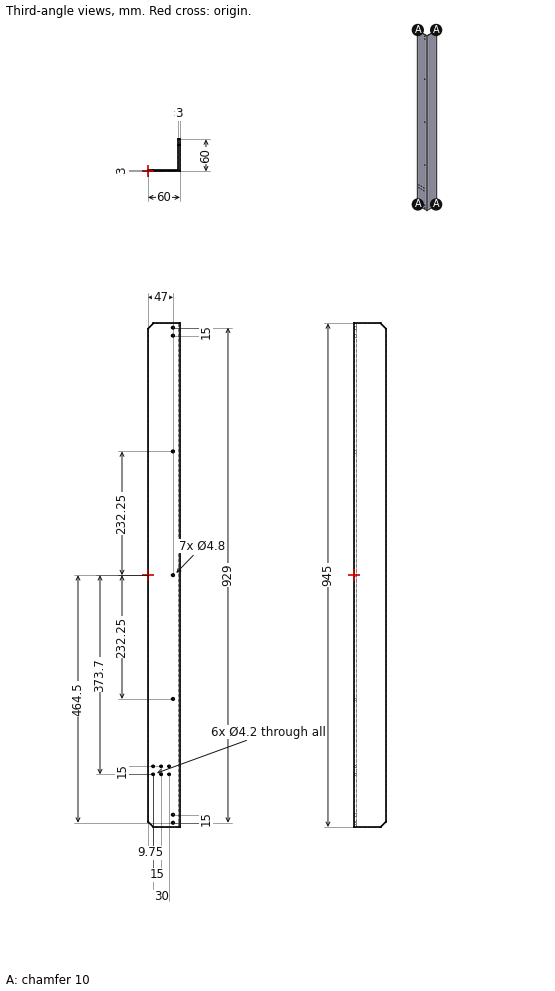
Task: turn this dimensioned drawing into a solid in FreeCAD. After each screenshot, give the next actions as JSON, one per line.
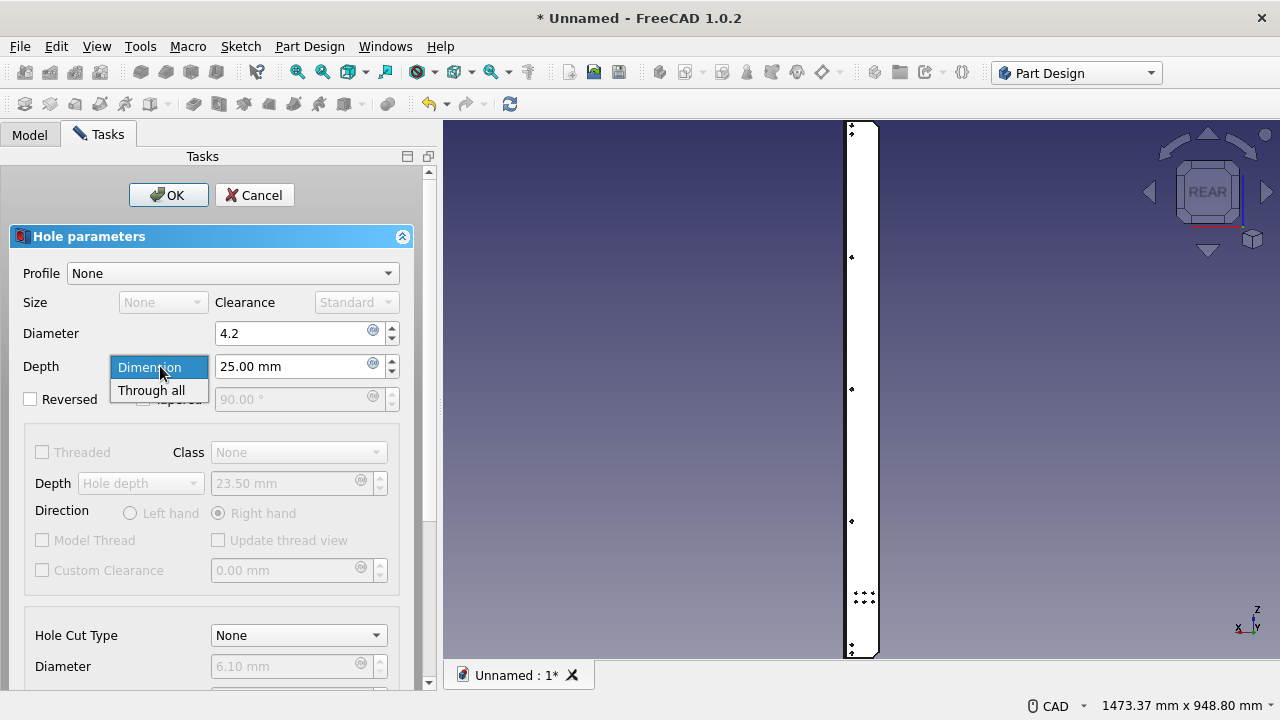
{"action": "left_click", "coordinate": [158, 390]}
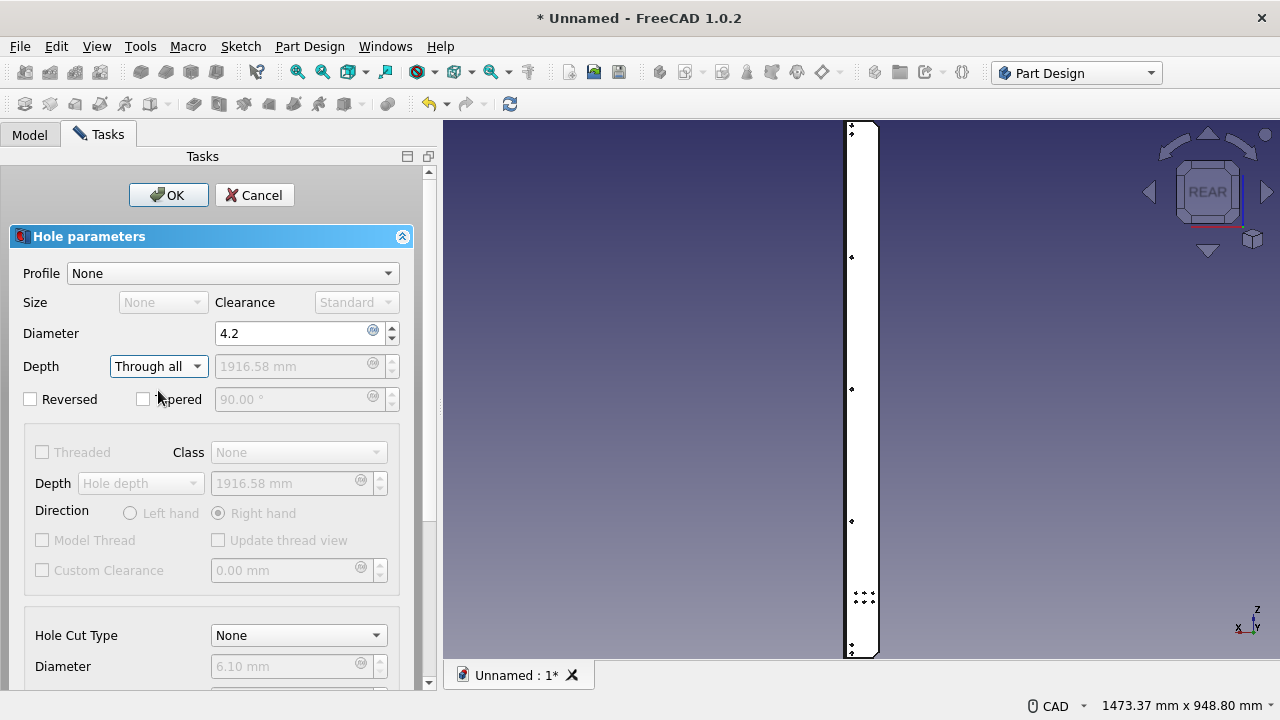
{"action": "left_click", "coordinate": [169, 195]}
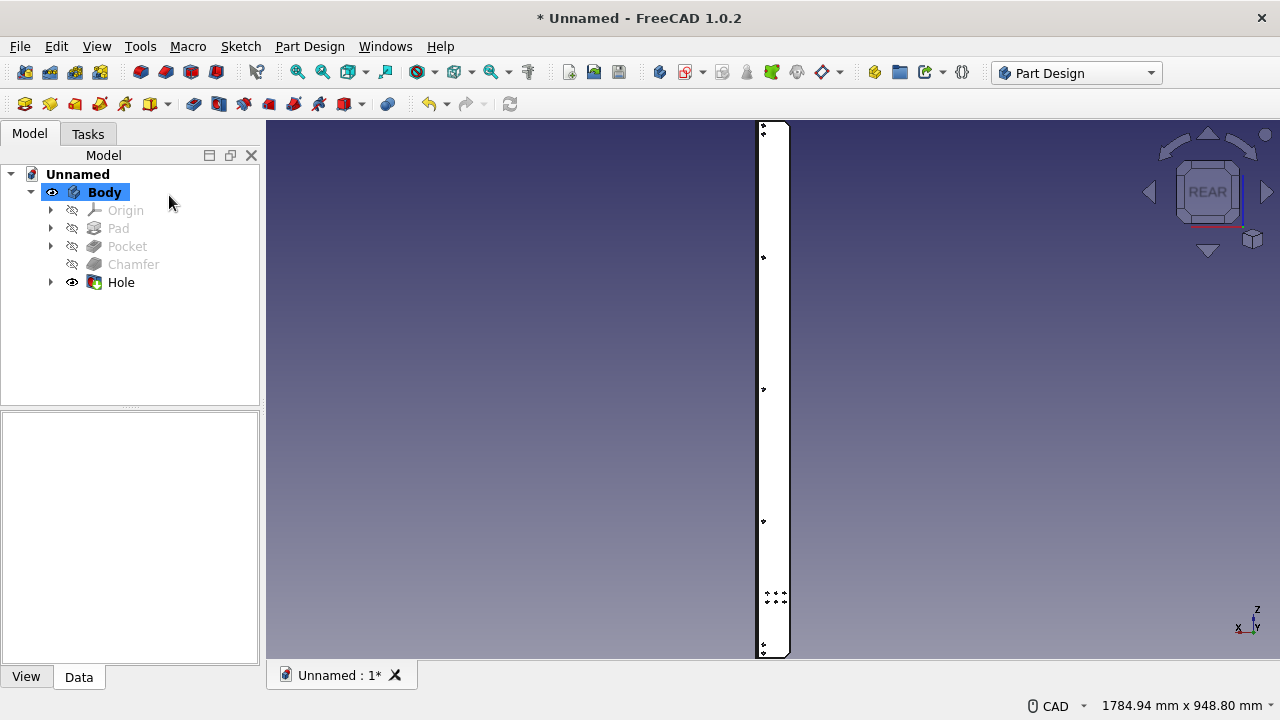
{"action": "key", "text": "0"}